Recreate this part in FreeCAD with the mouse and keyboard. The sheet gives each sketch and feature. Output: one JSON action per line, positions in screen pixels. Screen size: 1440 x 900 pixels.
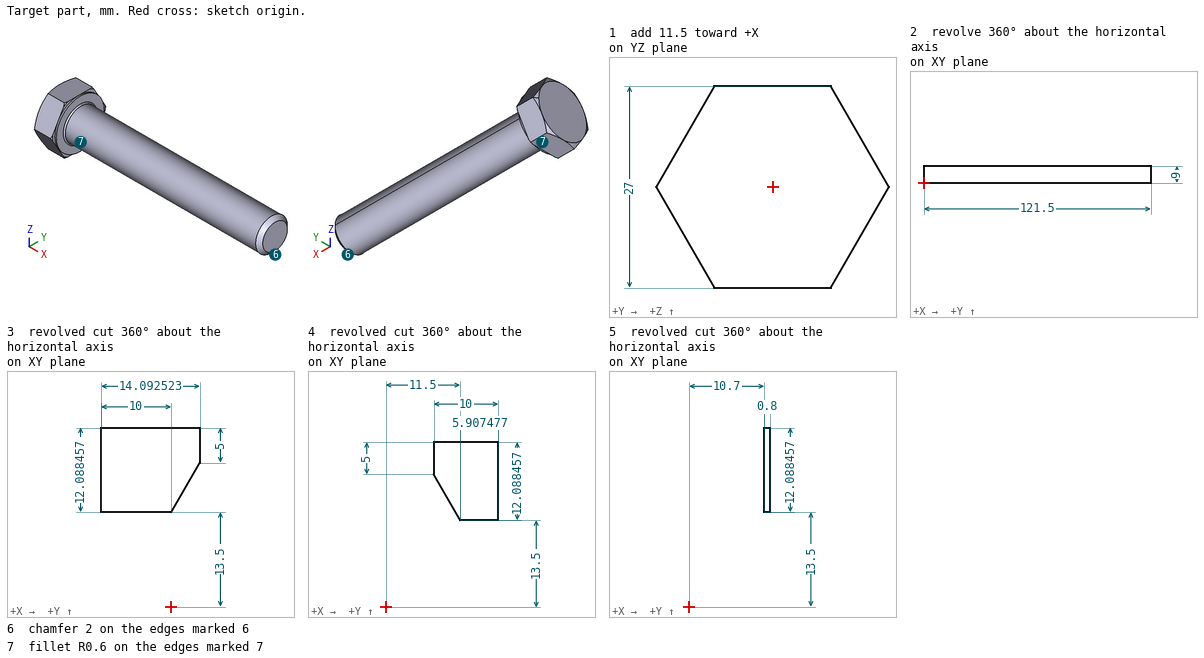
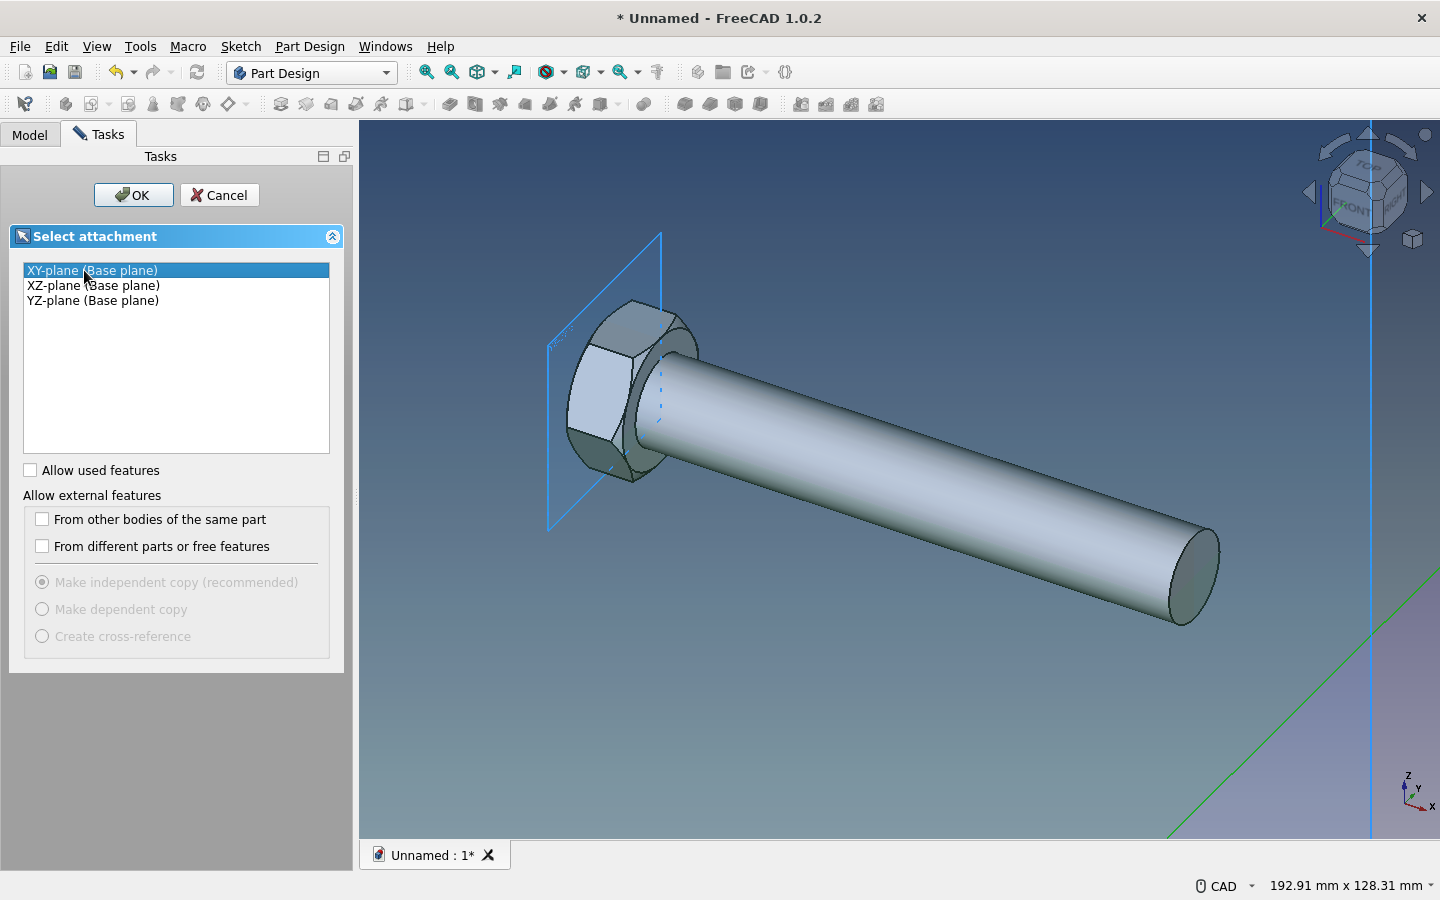
{"action": "left_click", "coordinate": [134, 195]}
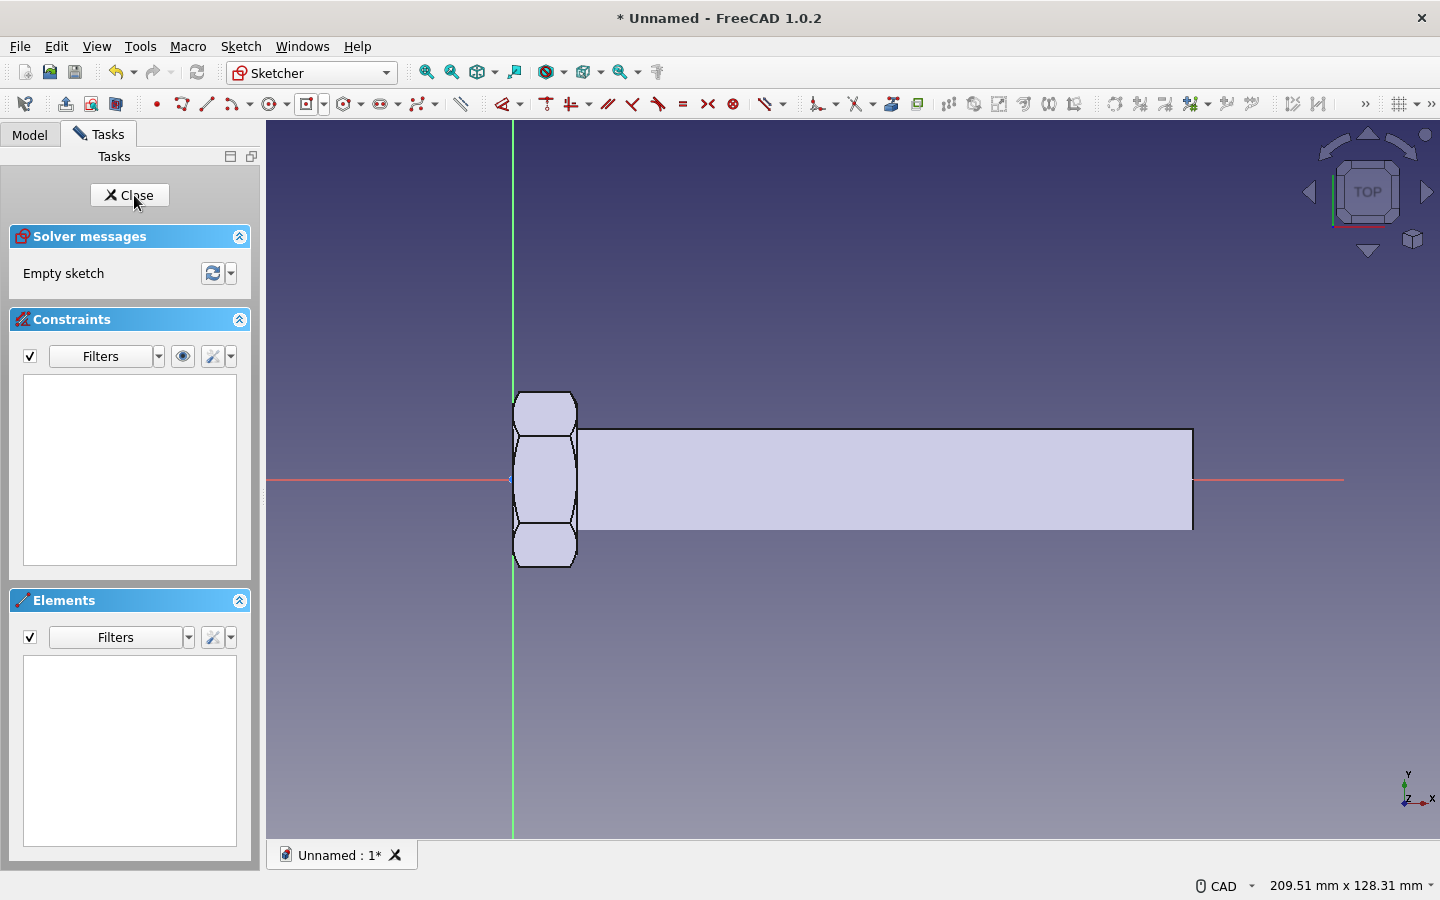
{"action": "left_click", "coordinate": [116, 104]}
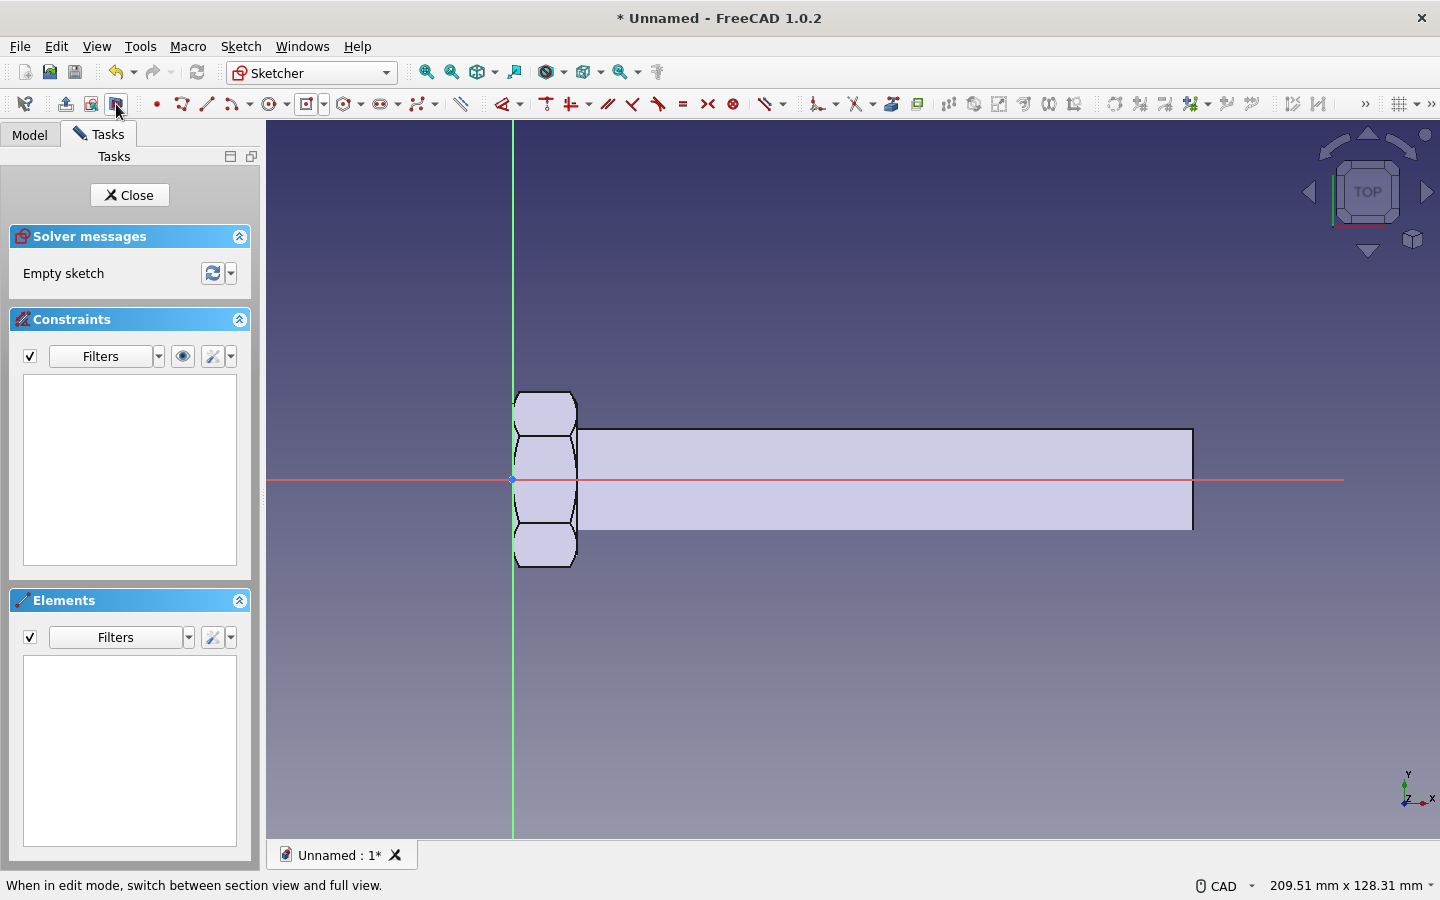
{"action": "scroll", "coordinate": [441, 377], "scroll_direction": "up", "scroll_amount": 6}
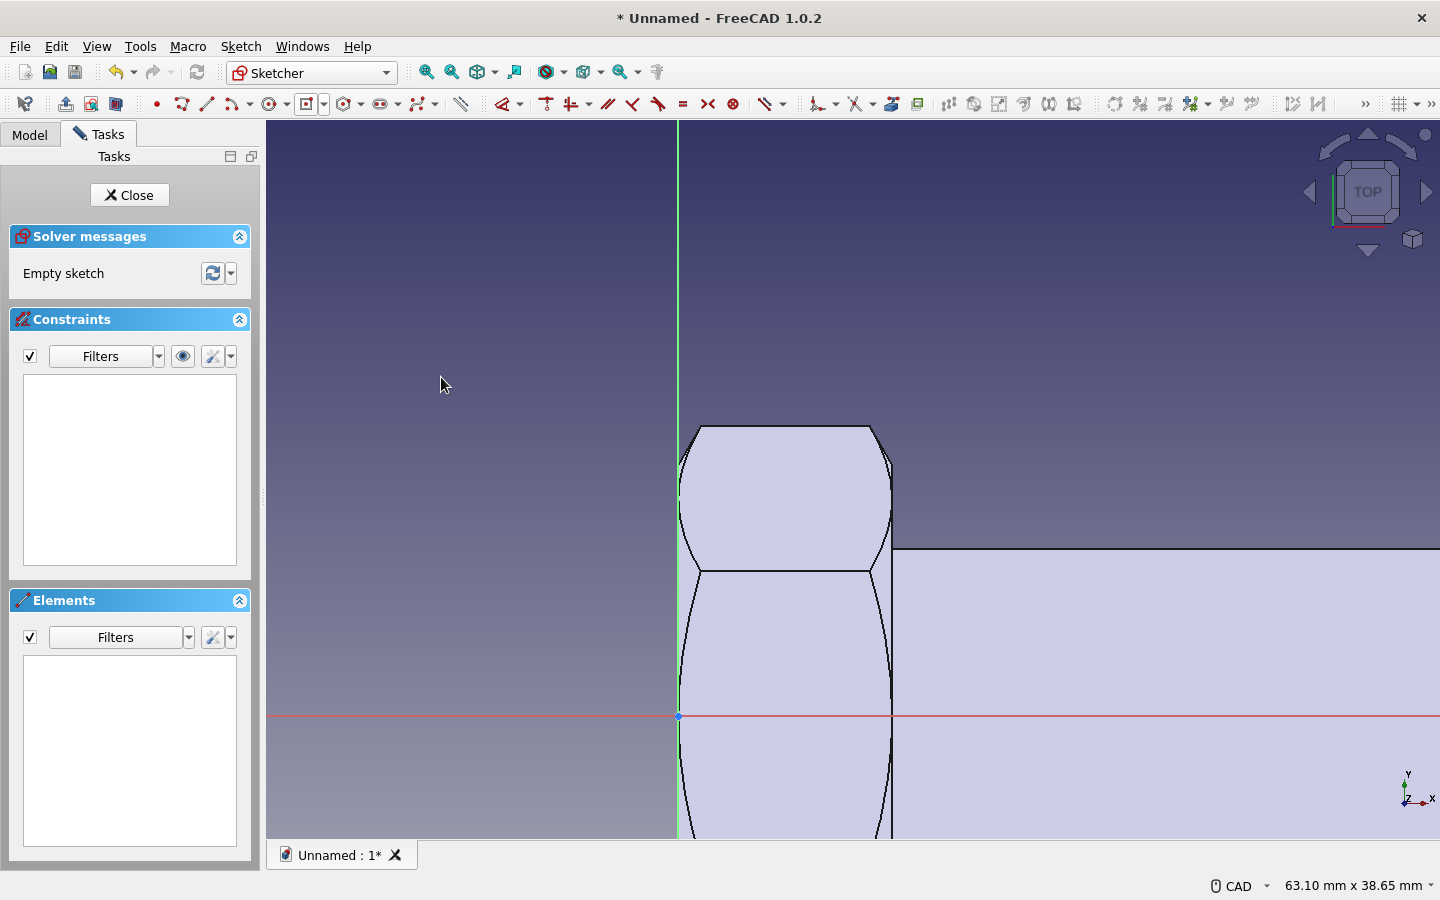
{"action": "left_click", "coordinate": [324, 104]}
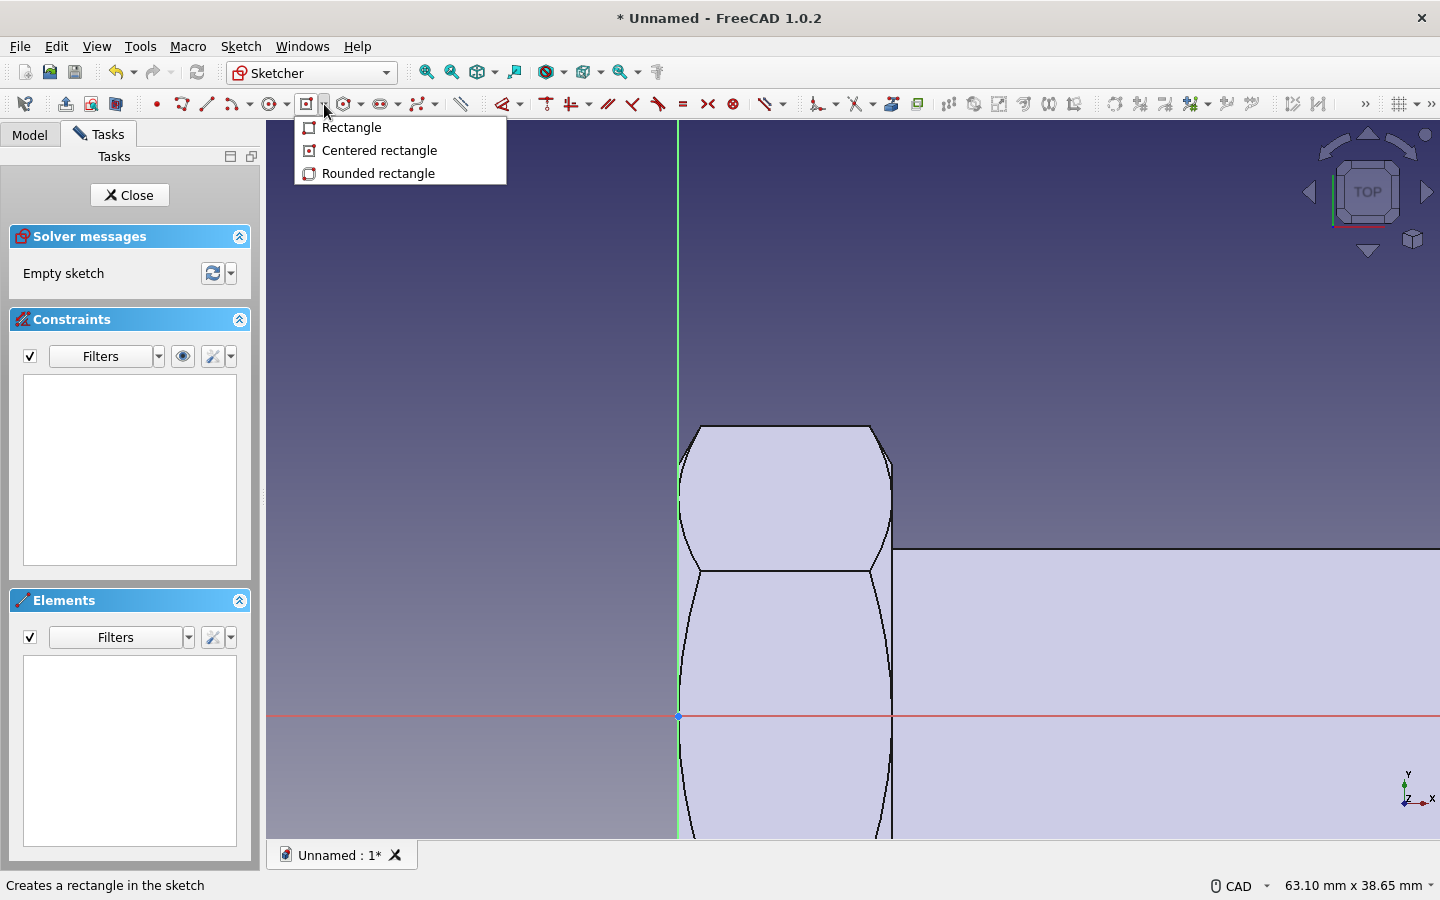
{"action": "left_click", "coordinate": [400, 128]}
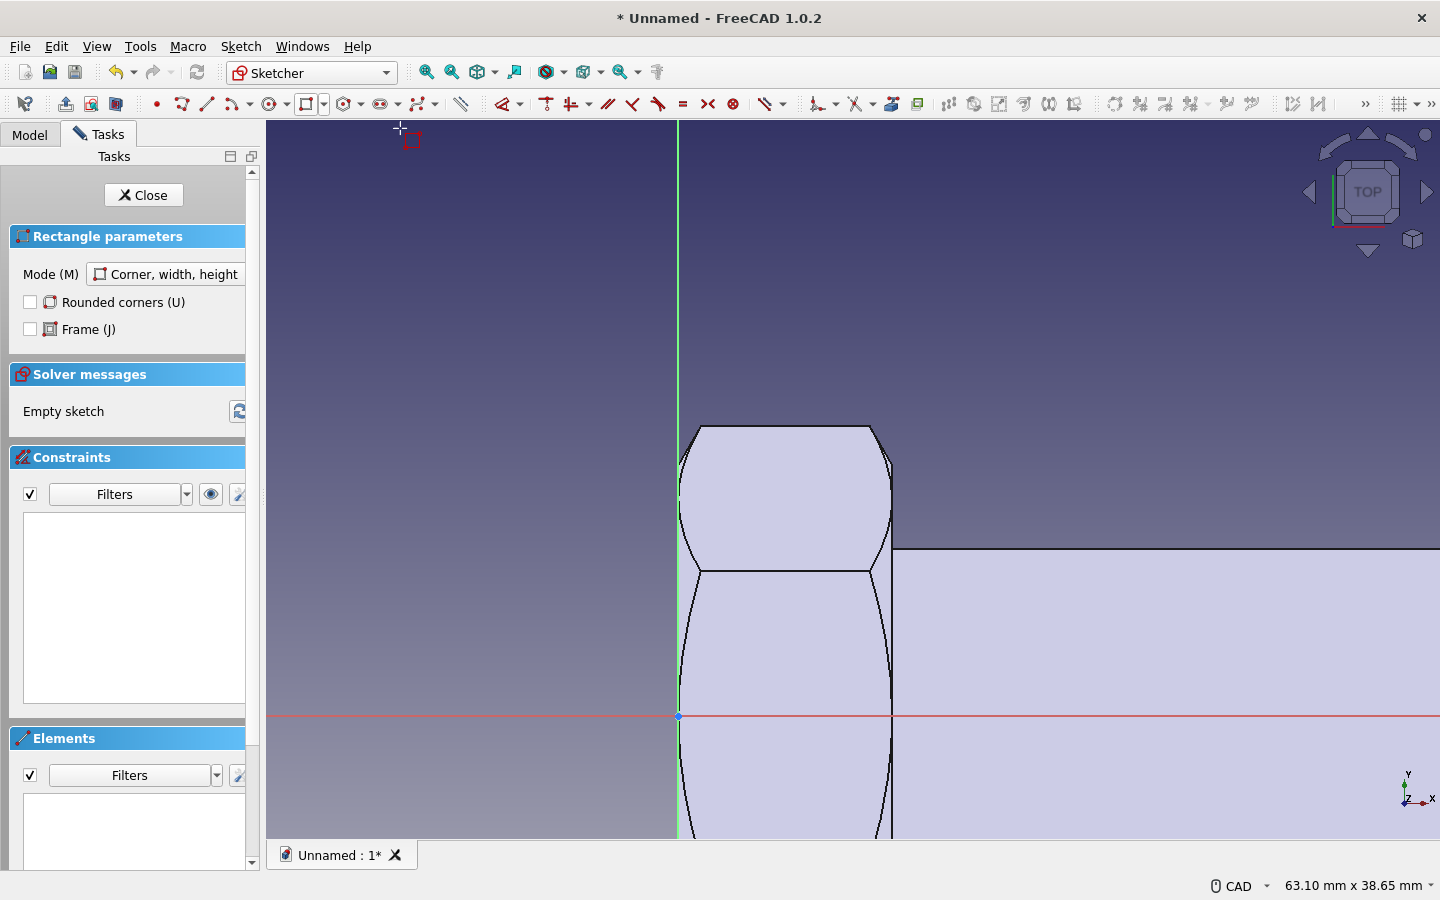
{"action": "left_click", "coordinate": [877, 240]}
{"action": "left_click", "coordinate": [892, 465]}
{"action": "key", "text": "Escape"}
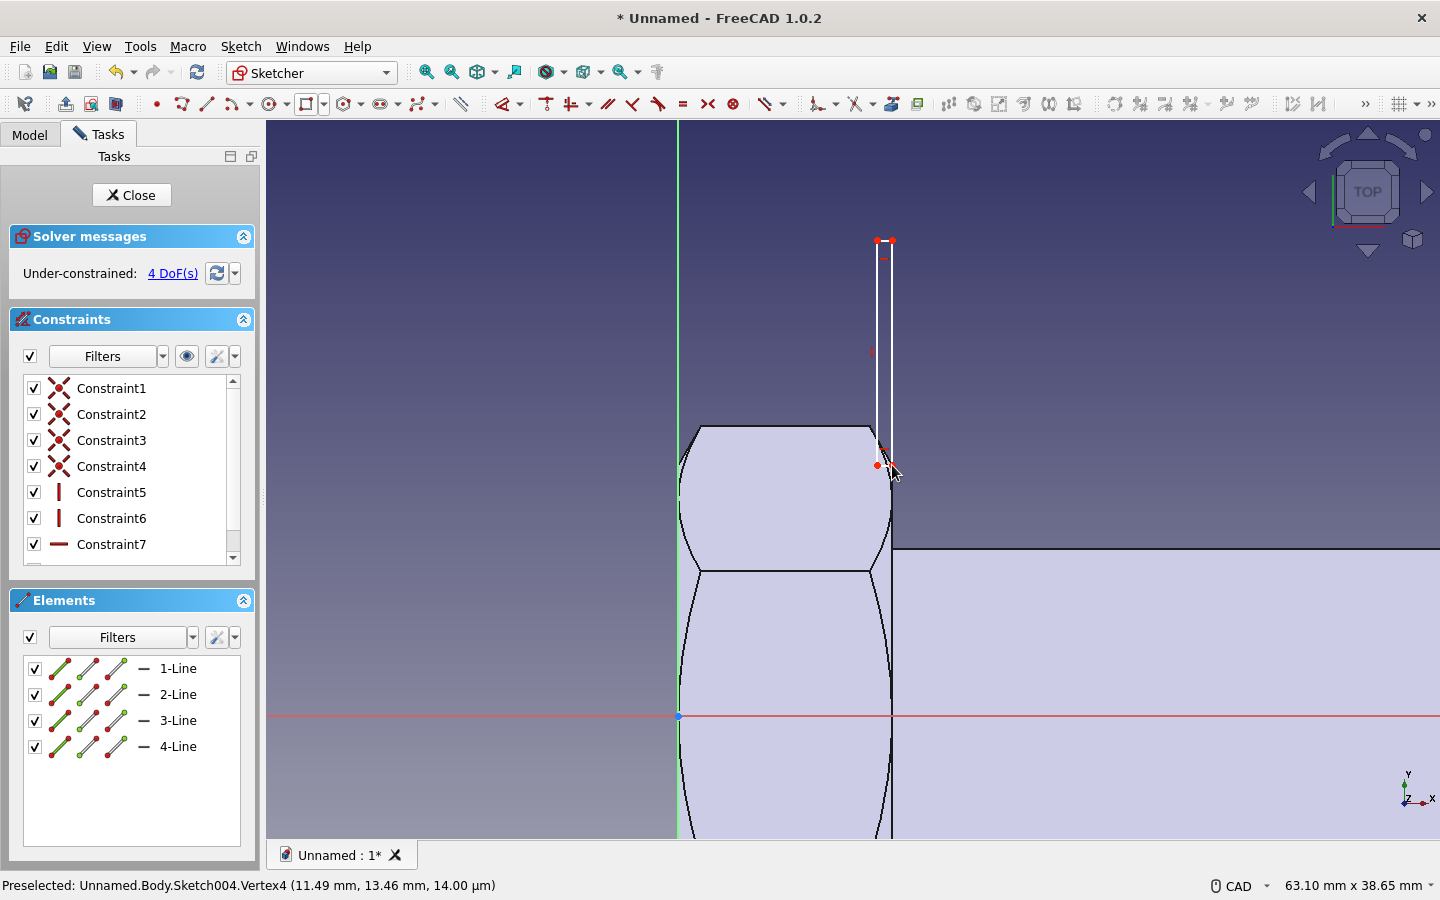
{"action": "left_click", "coordinate": [502, 104]}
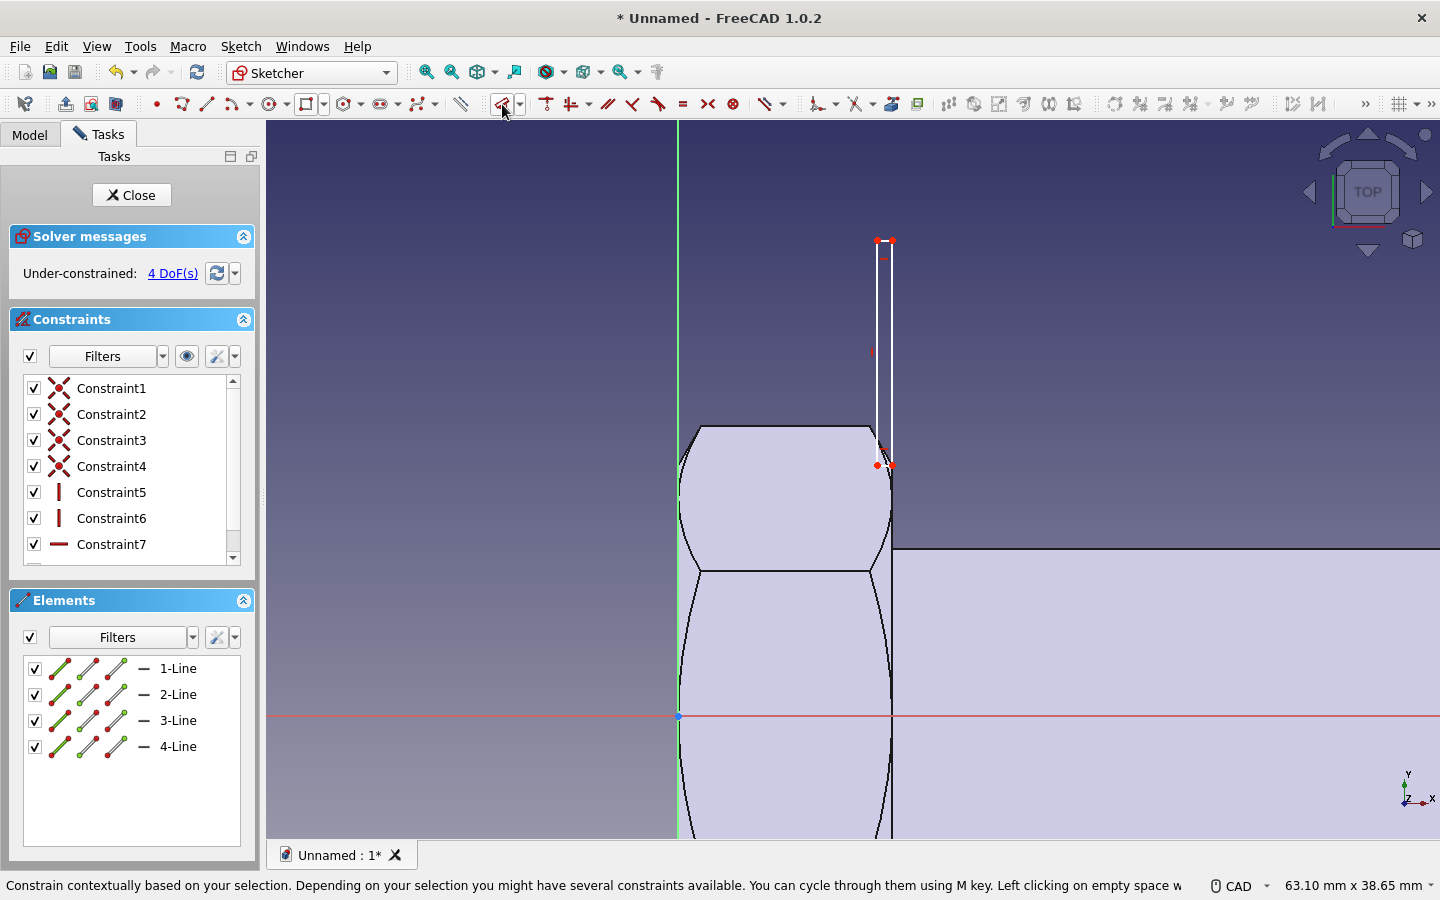
{"action": "scroll", "coordinate": [884, 466], "scroll_direction": "up", "scroll_amount": 5}